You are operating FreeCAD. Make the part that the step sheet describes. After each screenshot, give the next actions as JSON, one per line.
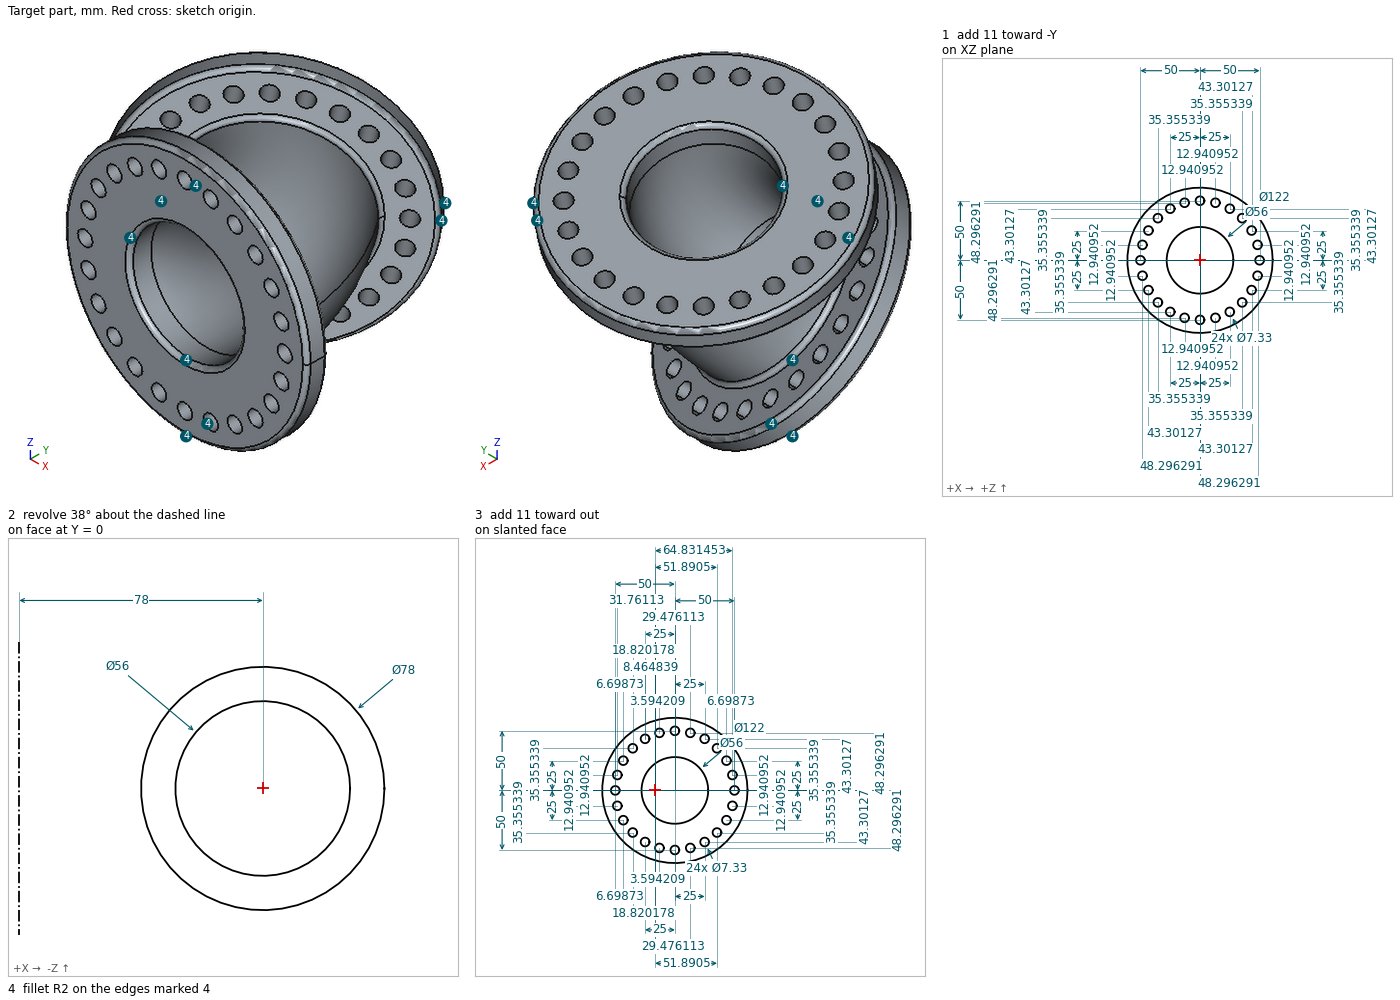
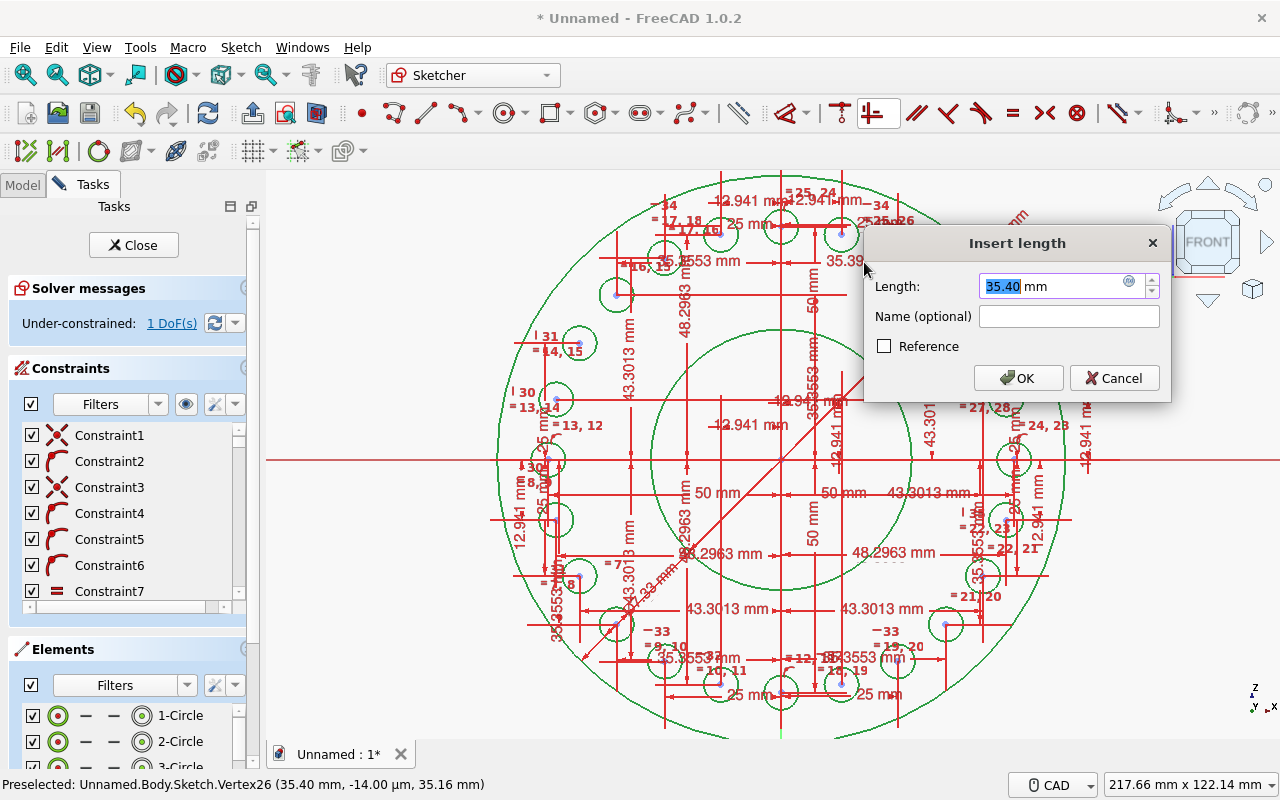
{"action": "type", "text": "35.355339"}
{"action": "key", "text": "Return"}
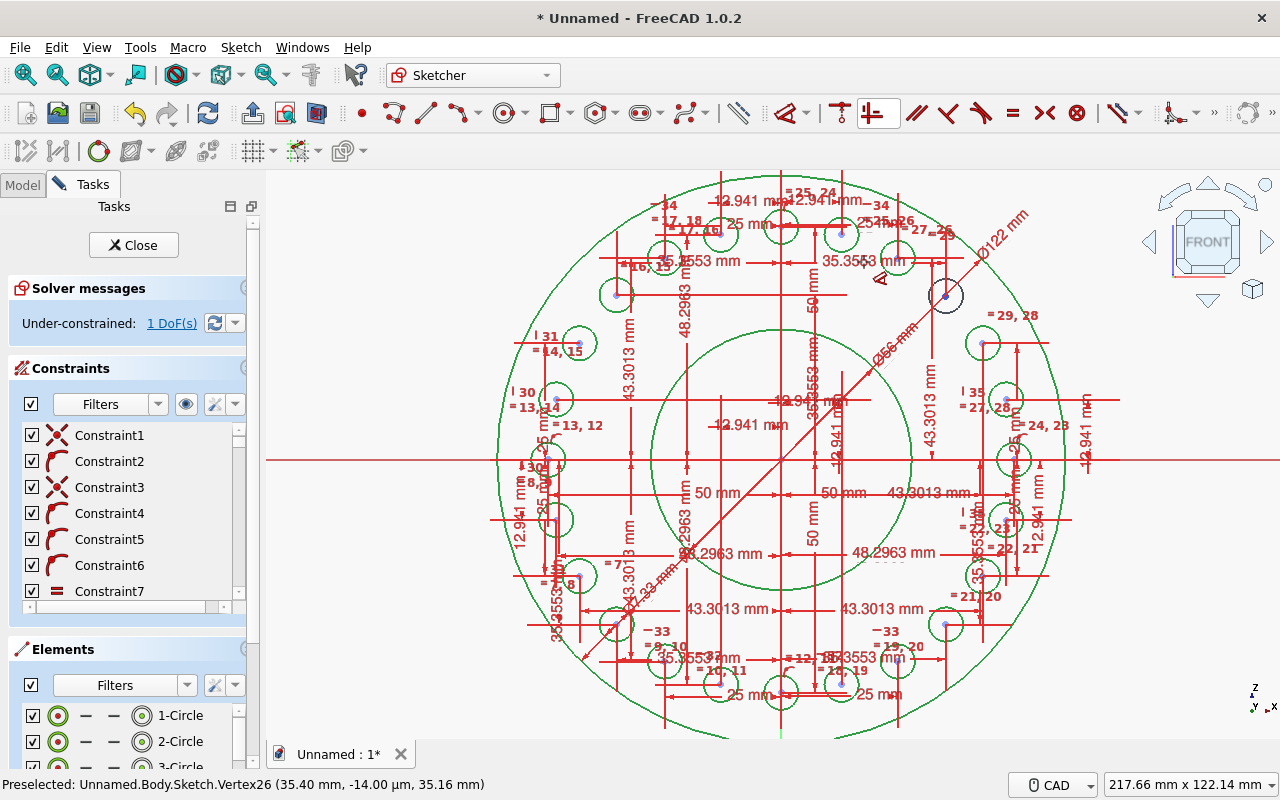
{"action": "left_click", "coordinate": [946, 296]}
{"action": "left_click", "coordinate": [980, 378]}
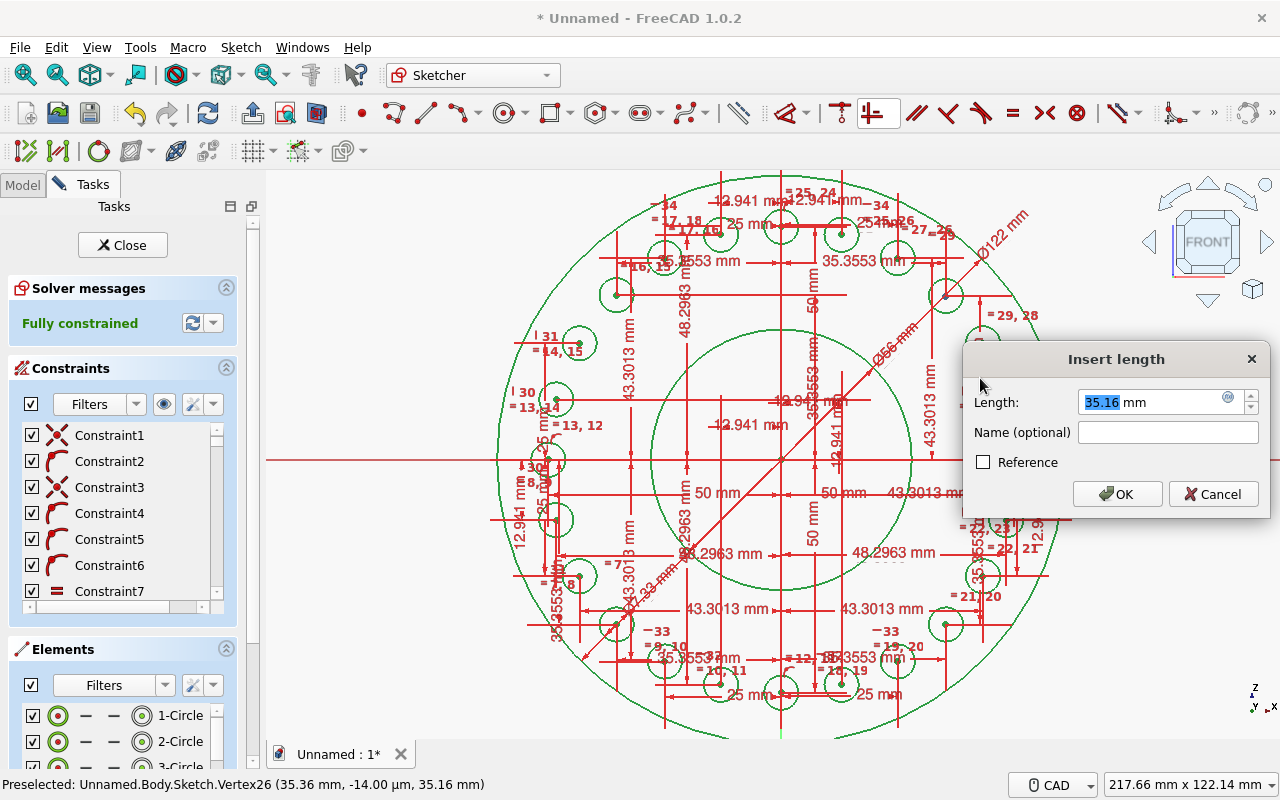
{"action": "type", "text": "35.355339"}
{"action": "key", "text": "Return"}
{"action": "key", "text": "Escape"}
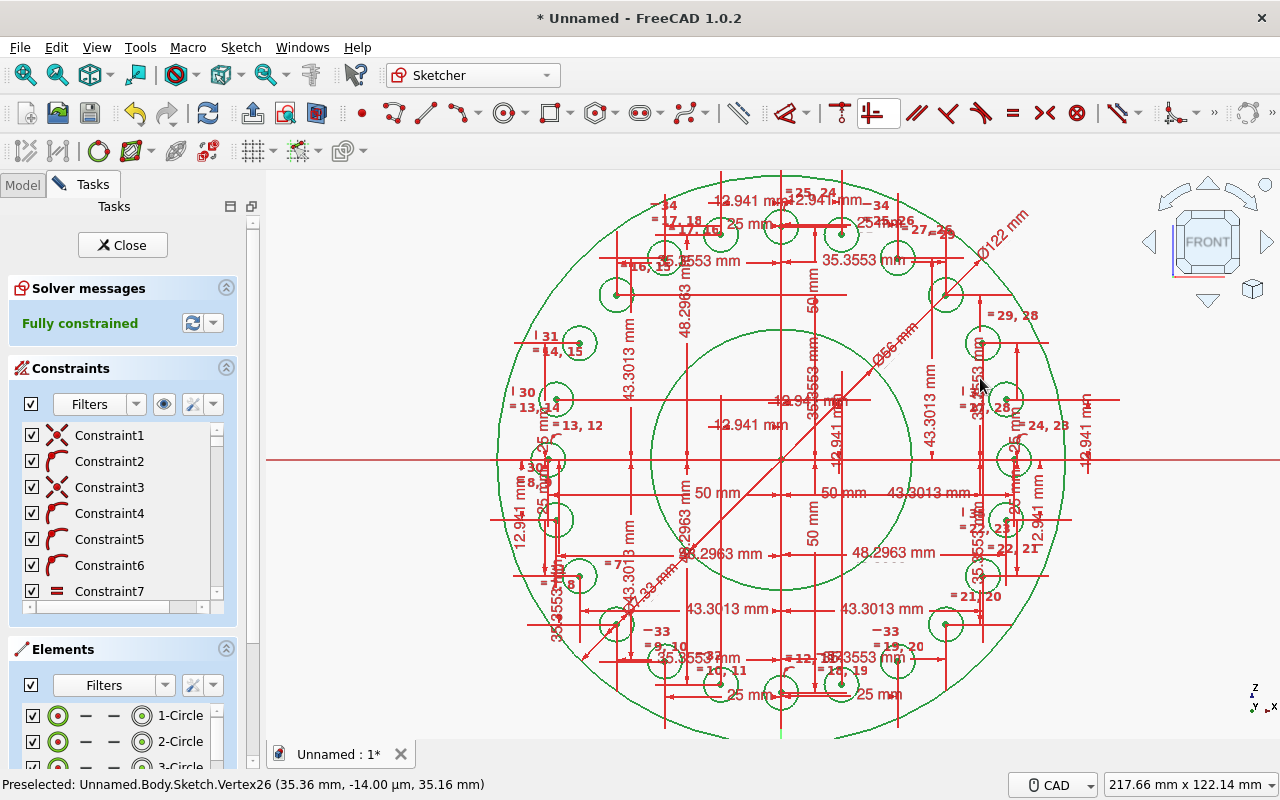
{"action": "left_click", "coordinate": [123, 245]}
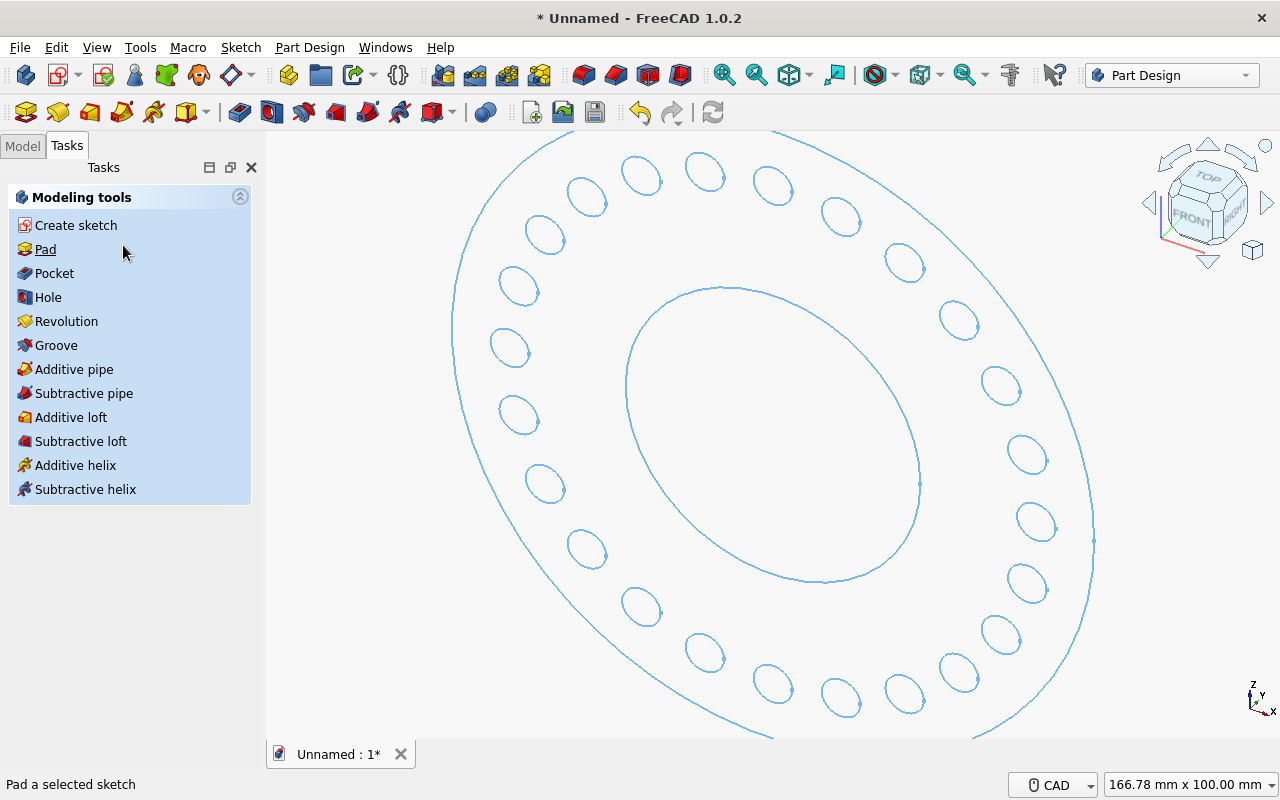
{"action": "left_click", "coordinate": [26, 112]}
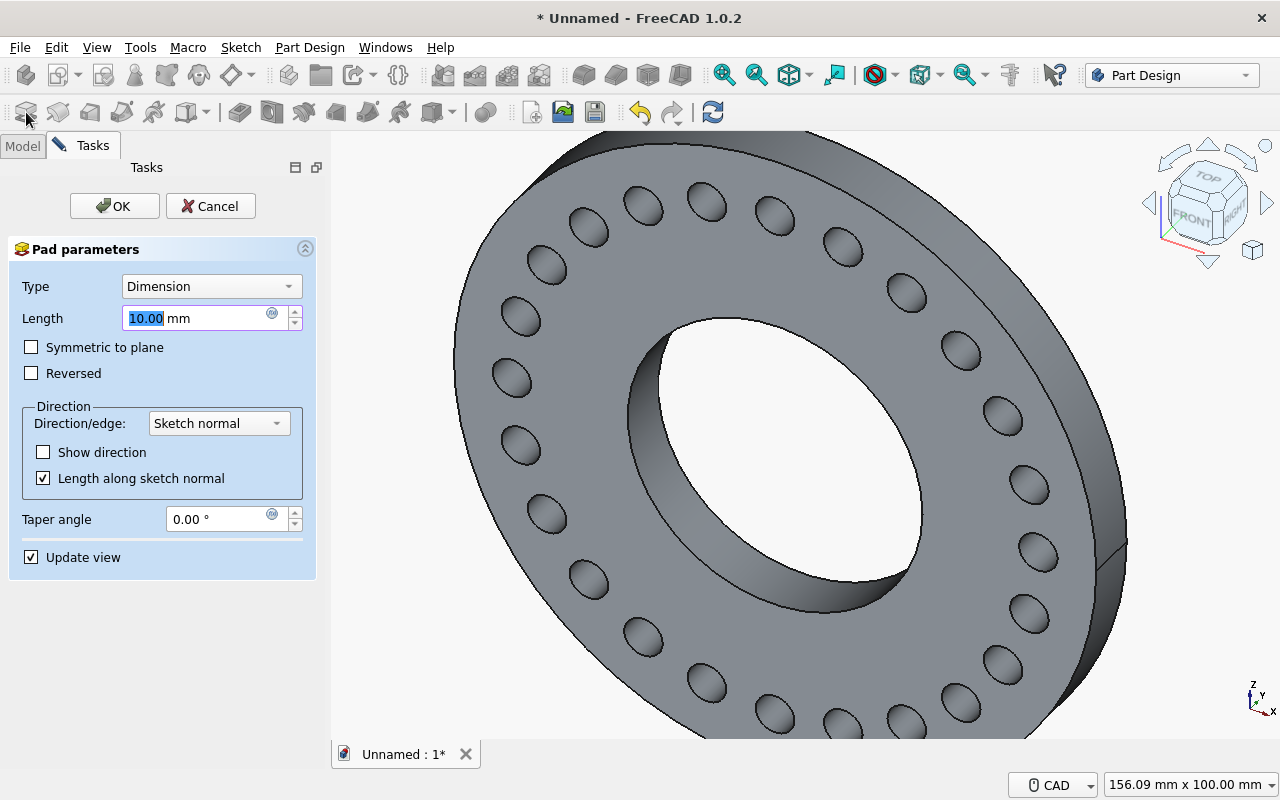
{"action": "type", "text": "11"}
{"action": "key", "text": "Tab"}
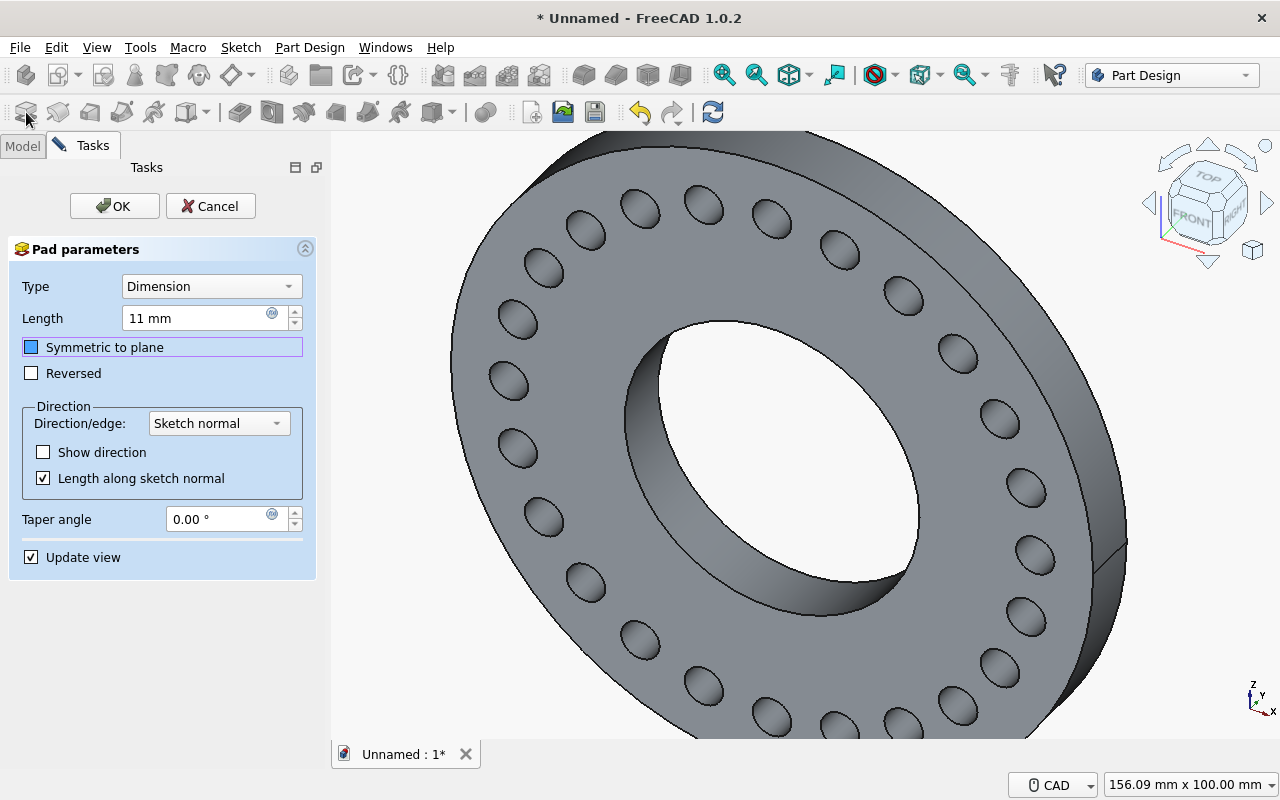
{"action": "left_click", "coordinate": [115, 206]}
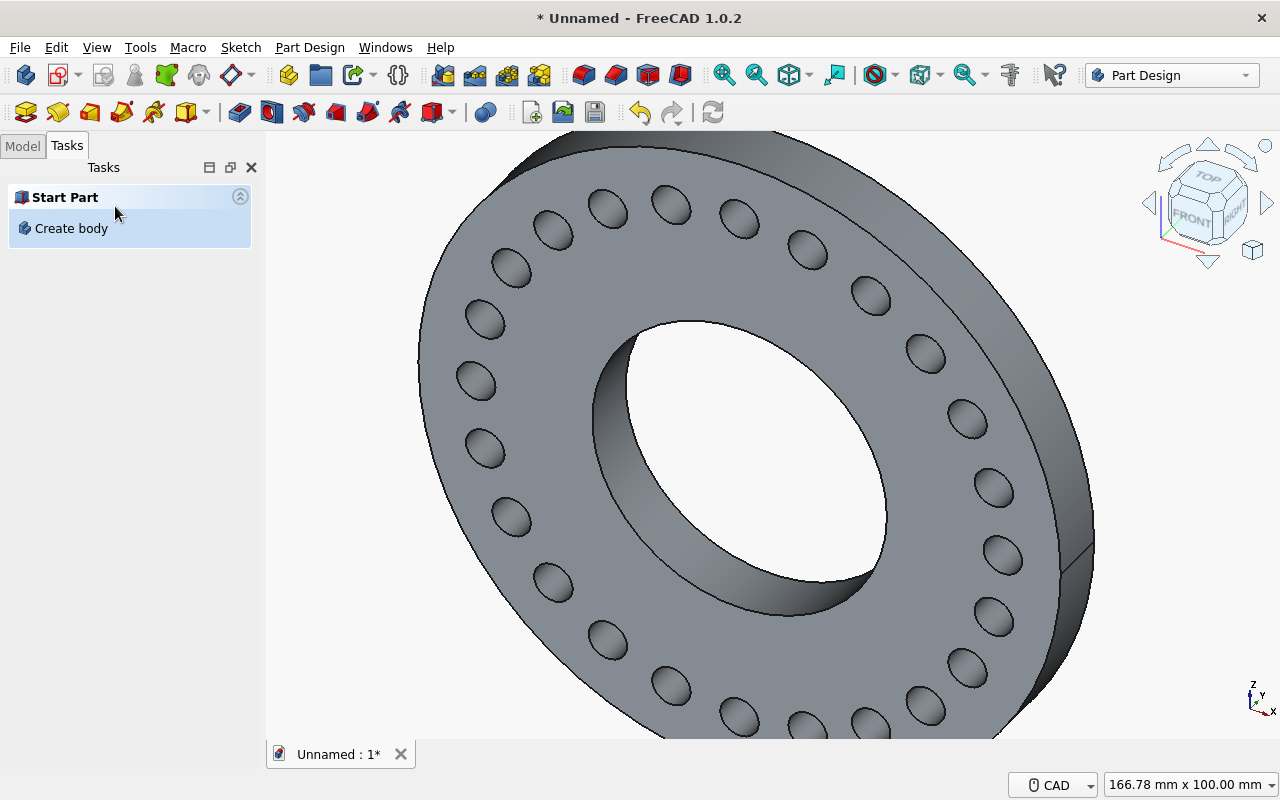
{"action": "left_click", "coordinate": [726, 76]}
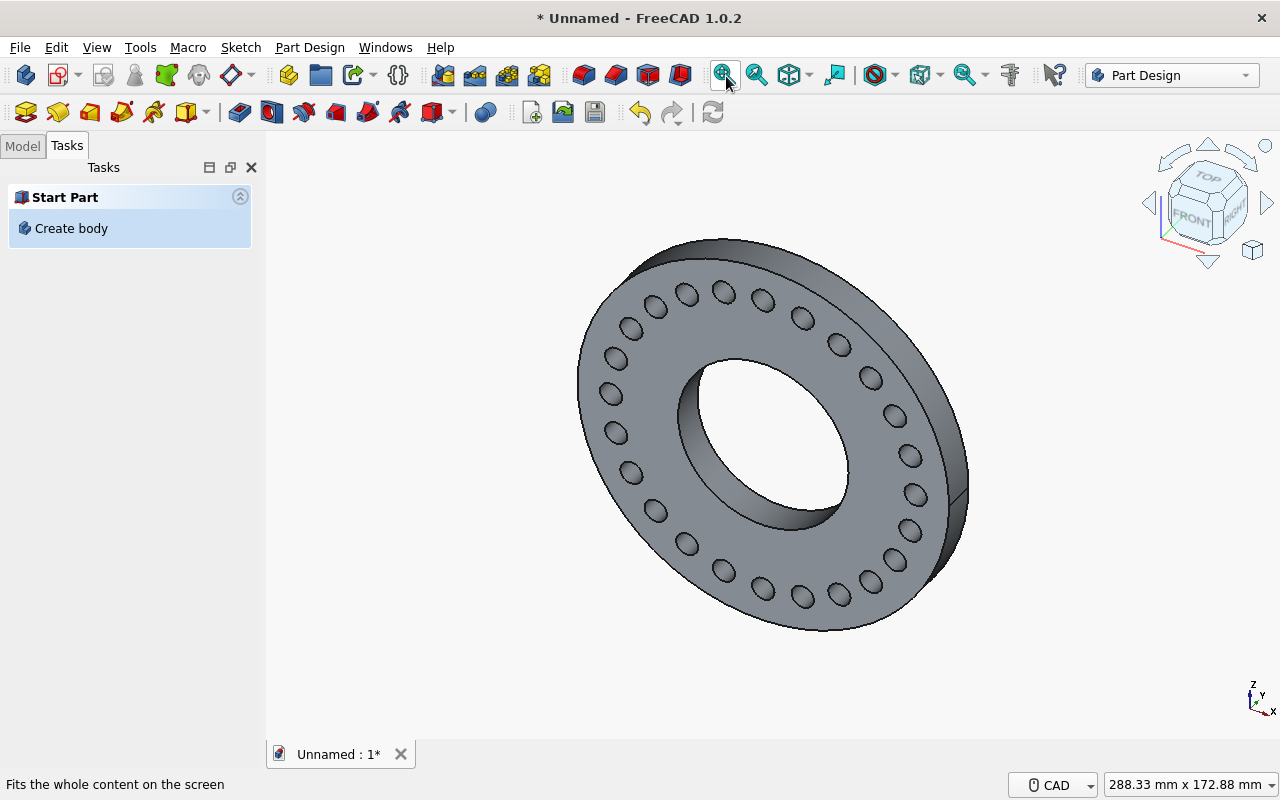
{"action": "key", "text": "4"}